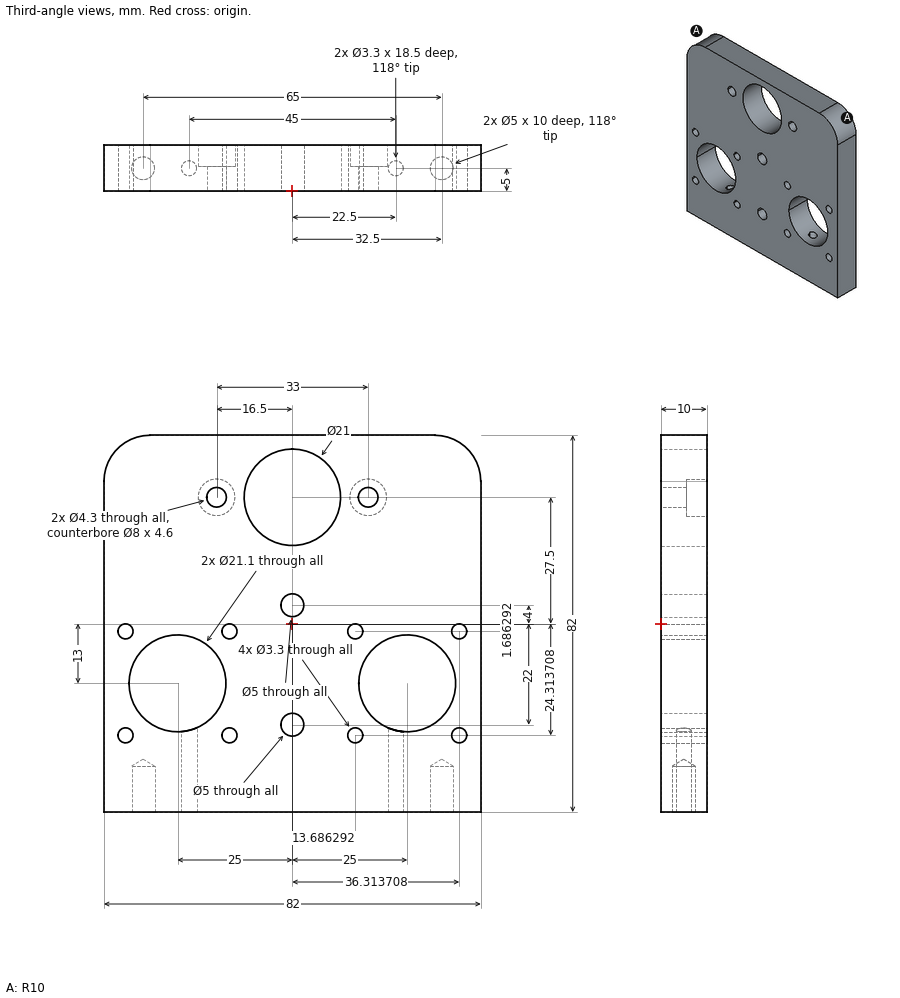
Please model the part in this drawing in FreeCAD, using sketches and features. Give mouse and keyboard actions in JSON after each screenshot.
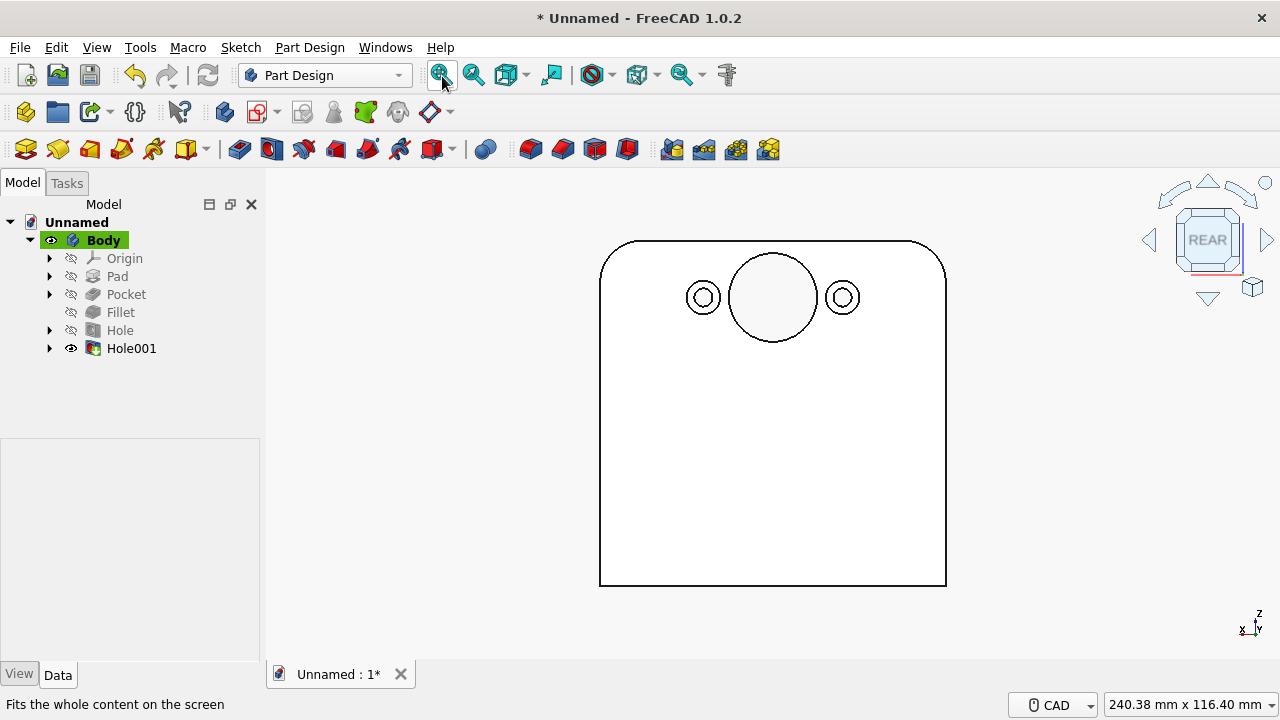
{"action": "left_click", "coordinate": [724, 462]}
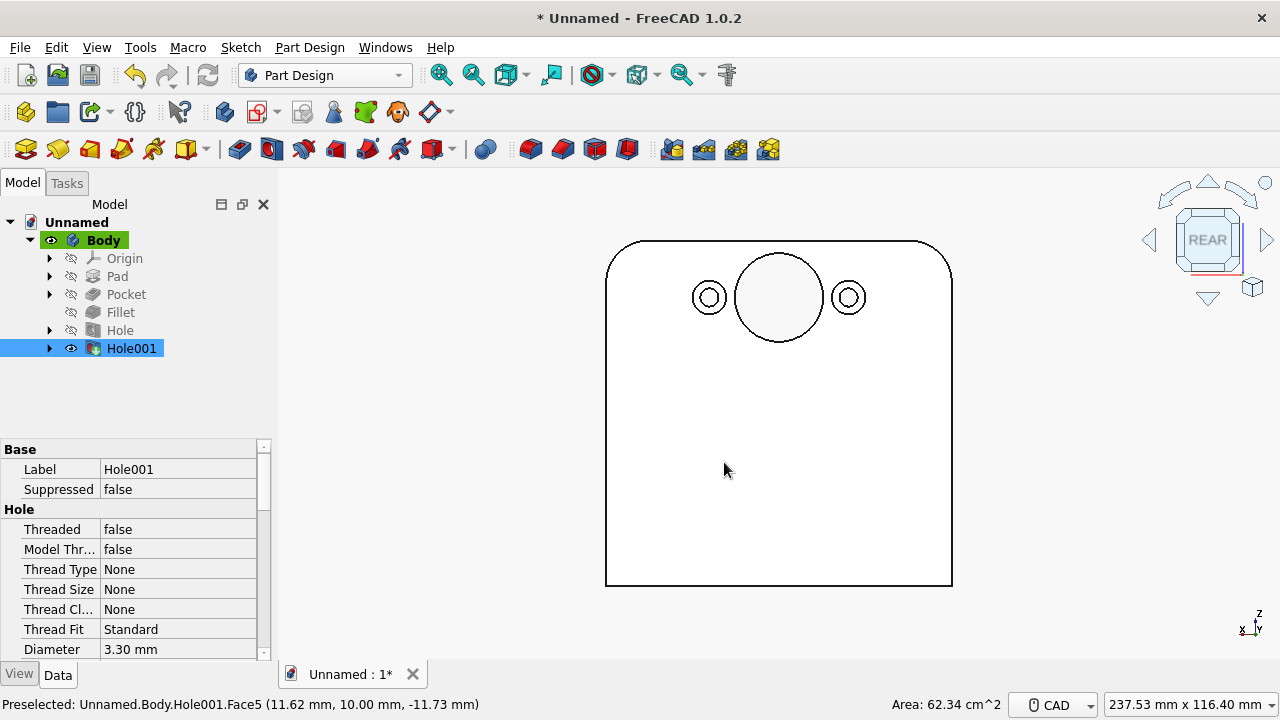
{"action": "left_click", "coordinate": [258, 112]}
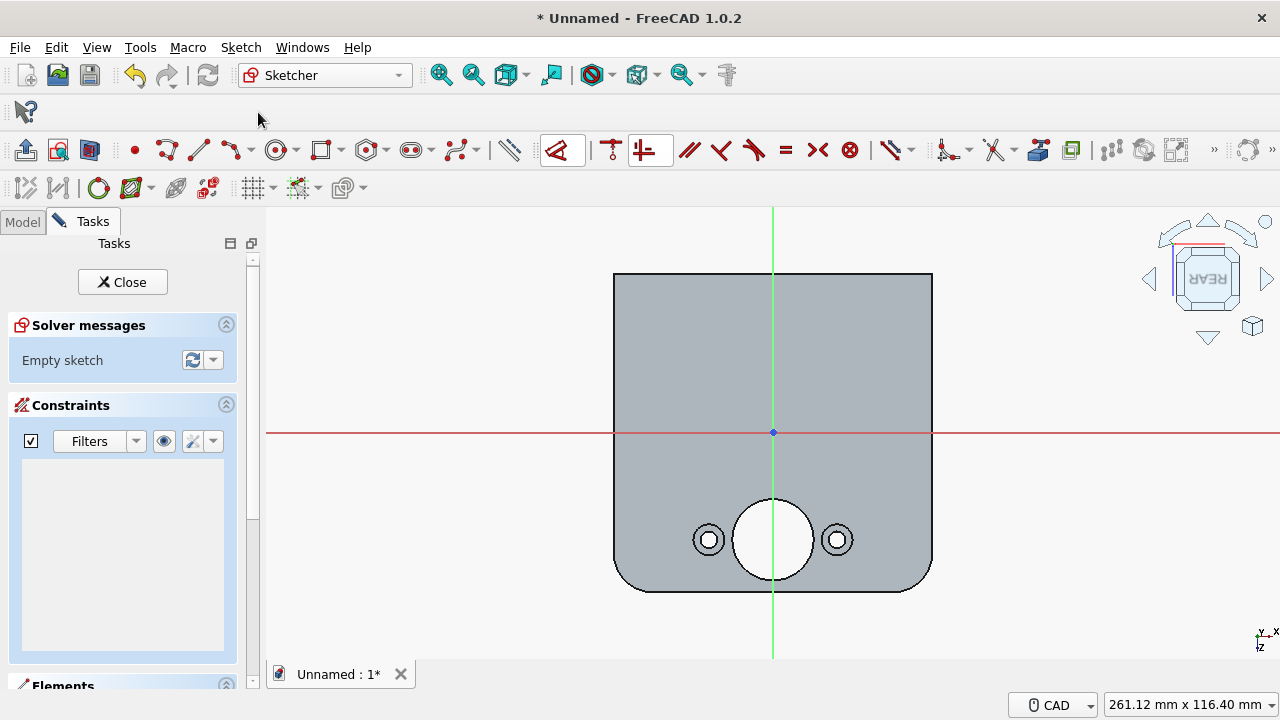
{"action": "scroll", "coordinate": [829, 350], "scroll_direction": "up", "scroll_amount": 4}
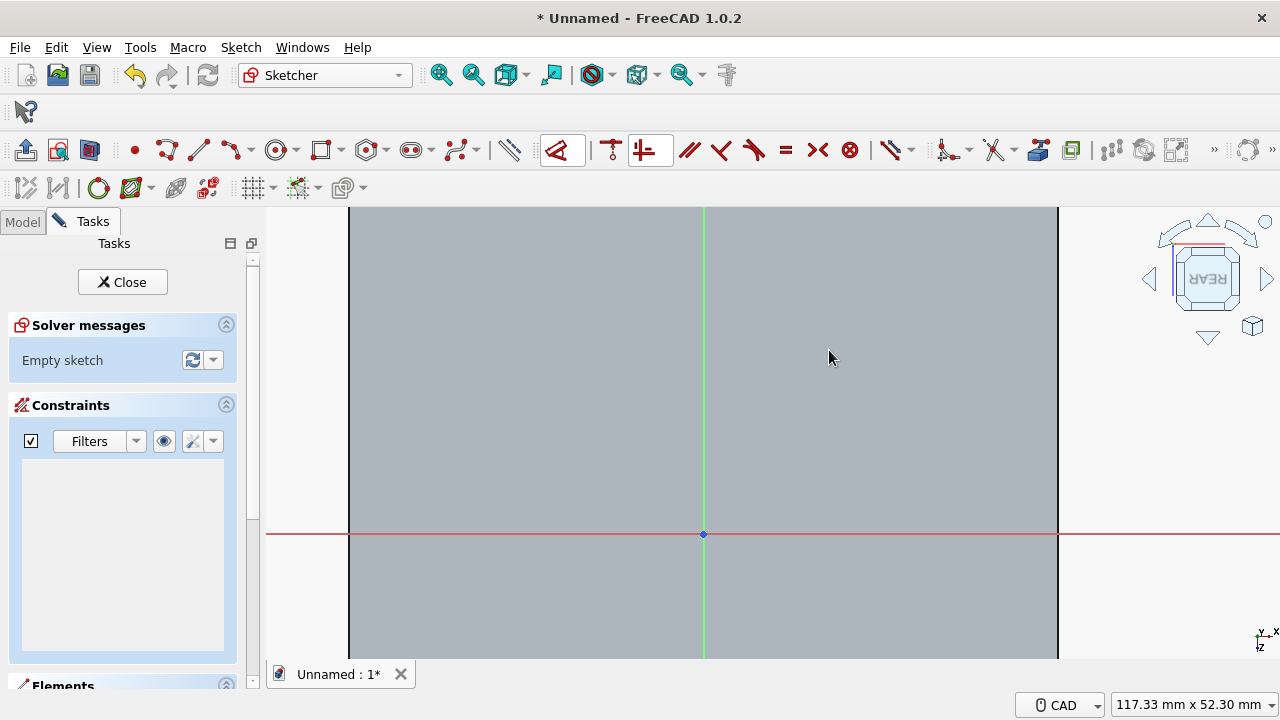
{"action": "left_click", "coordinate": [276, 150]}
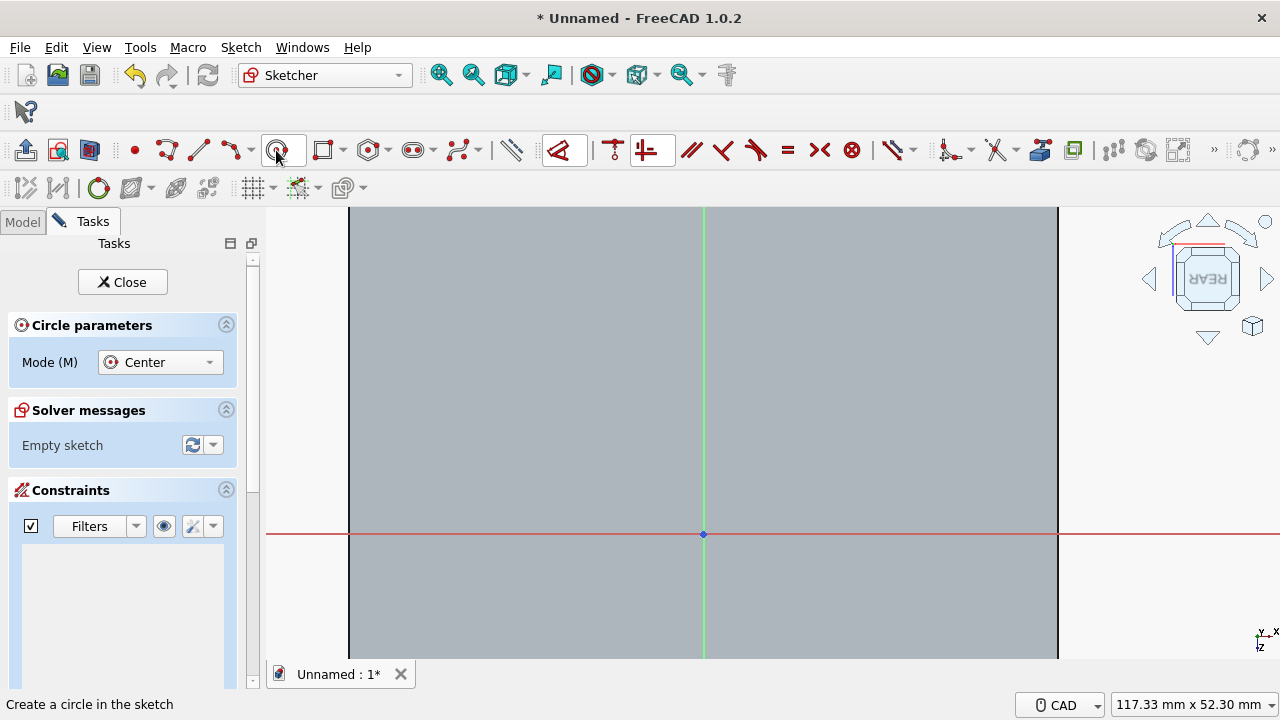
{"action": "left_click", "coordinate": [488, 422]}
{"action": "left_click", "coordinate": [552, 358]}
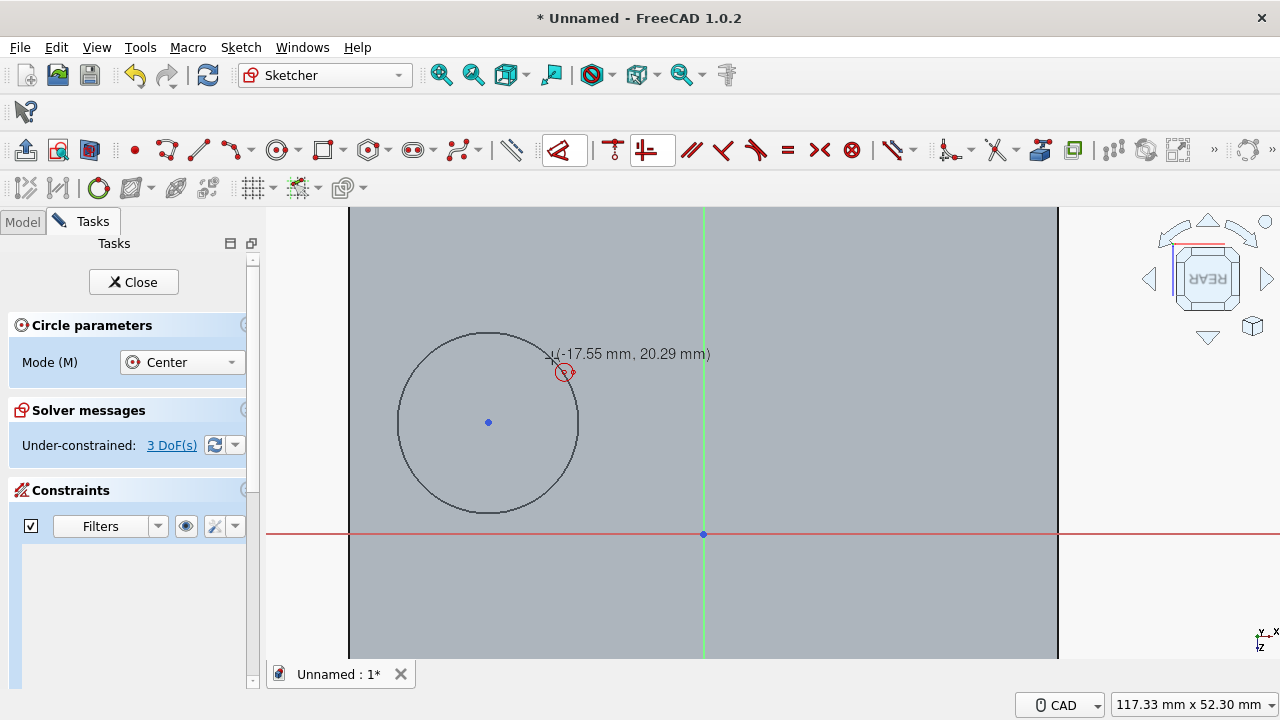
{"action": "left_click", "coordinate": [920, 422]}
{"action": "left_click", "coordinate": [984, 358]}
{"action": "key", "text": "Escape"}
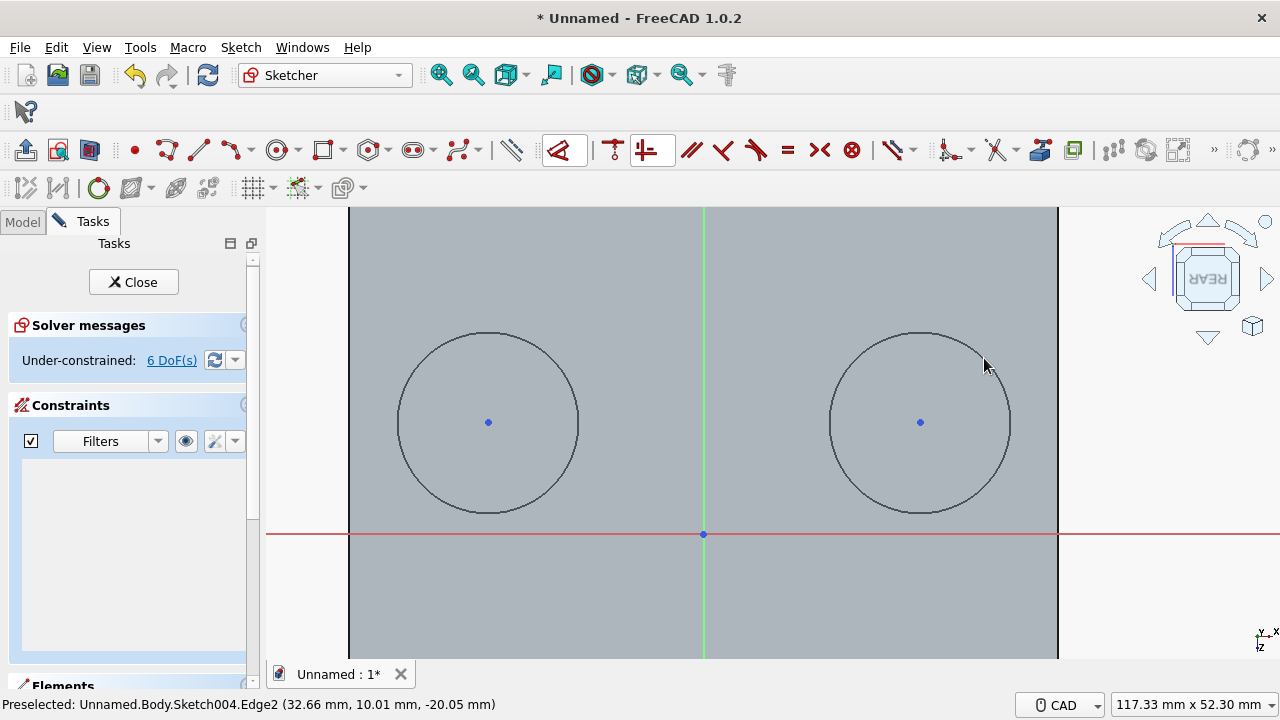
{"action": "left_click", "coordinate": [552, 359]}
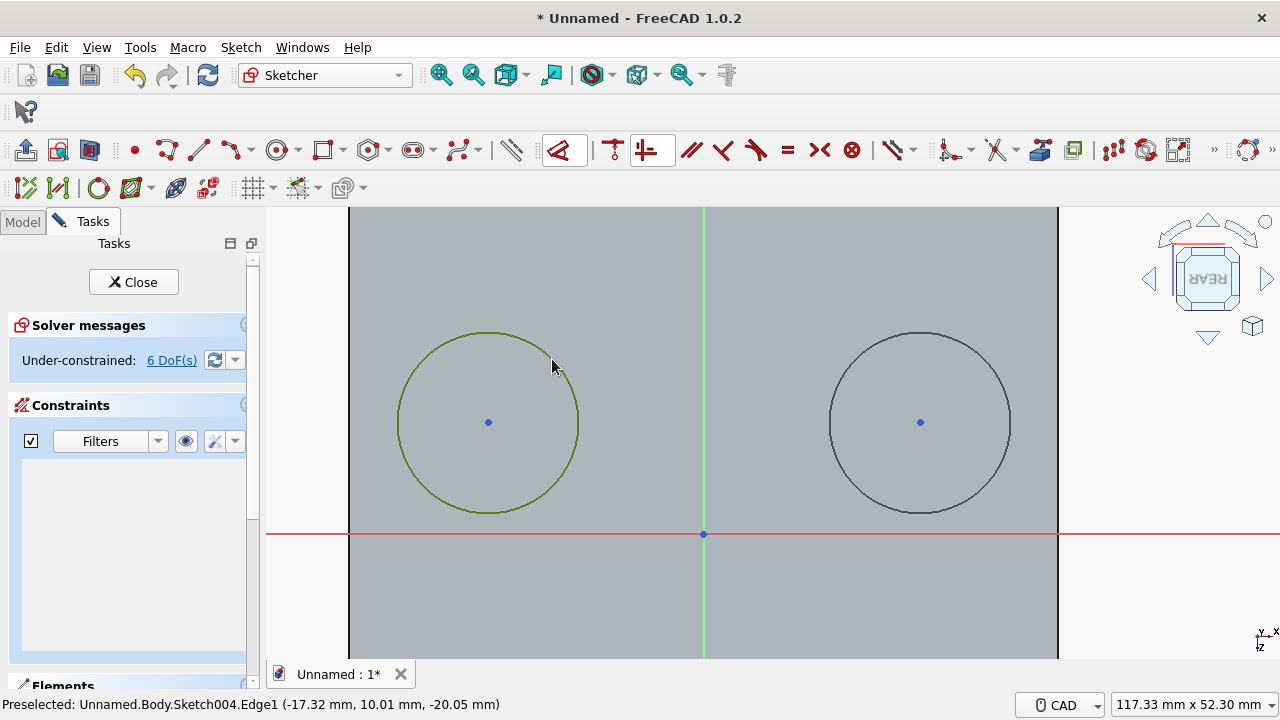
{"action": "left_click", "coordinate": [984, 359]}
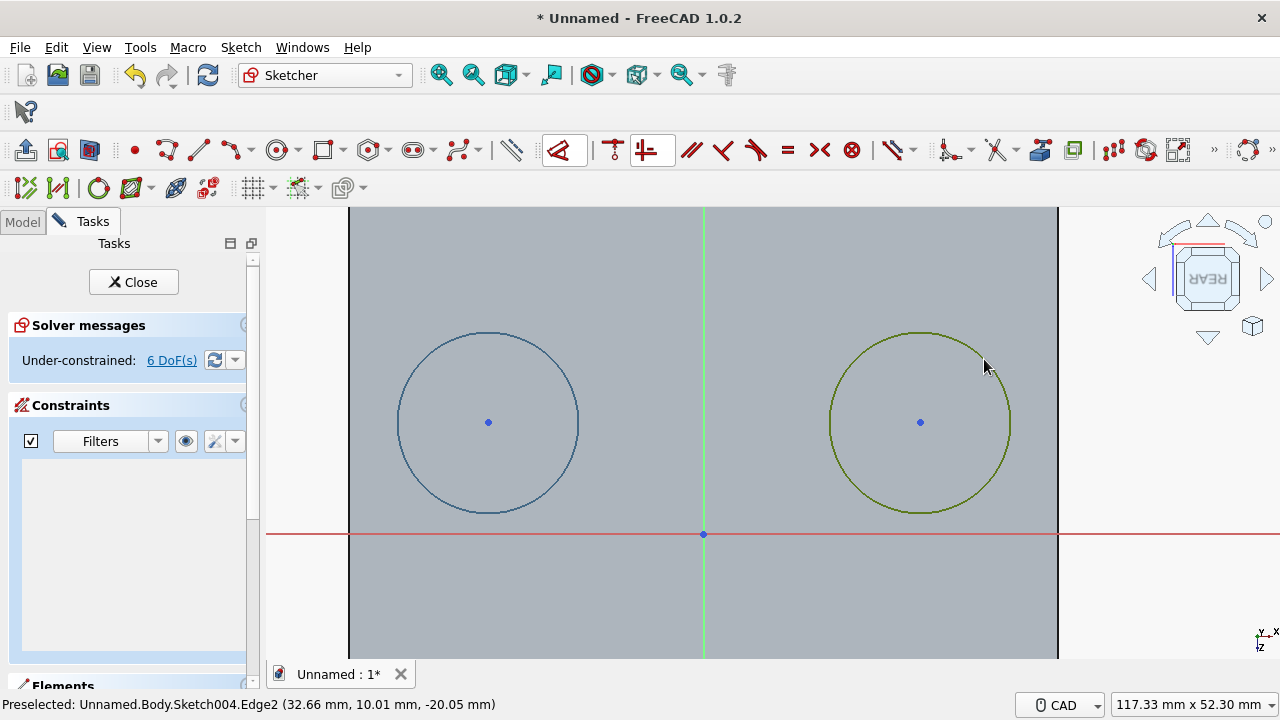
{"action": "left_click", "coordinate": [788, 150]}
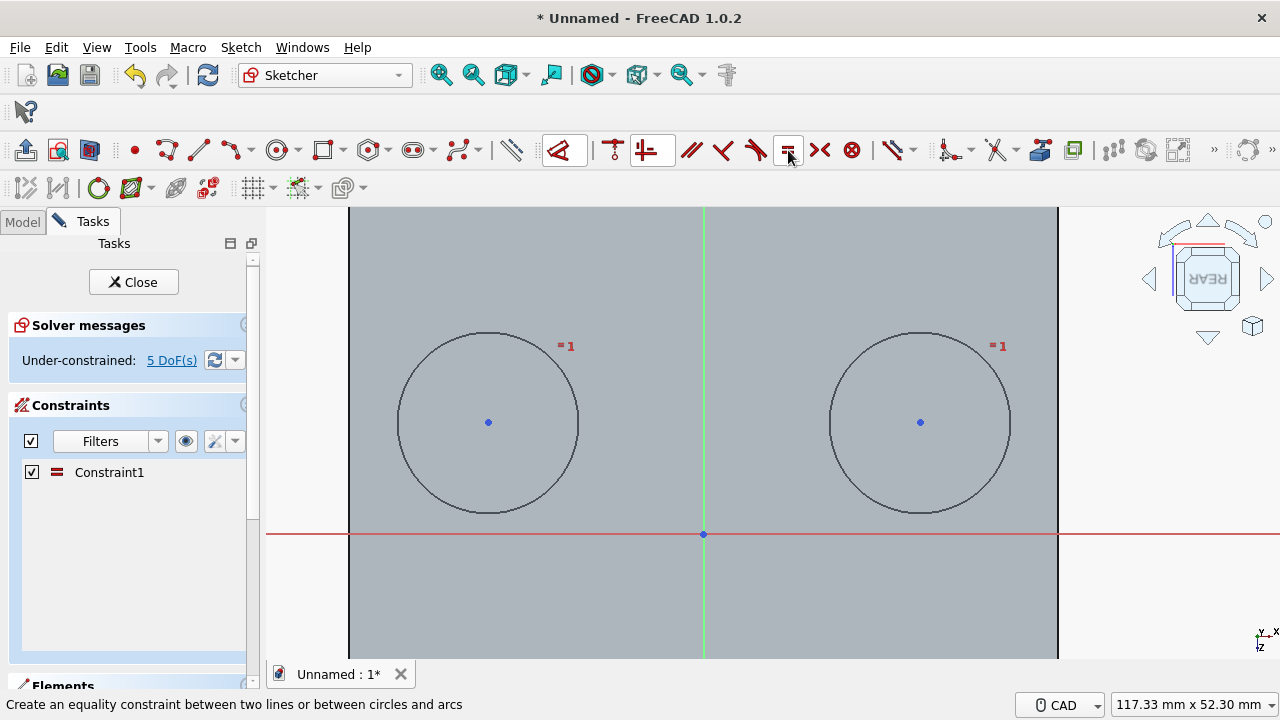
{"action": "left_click", "coordinate": [552, 359]}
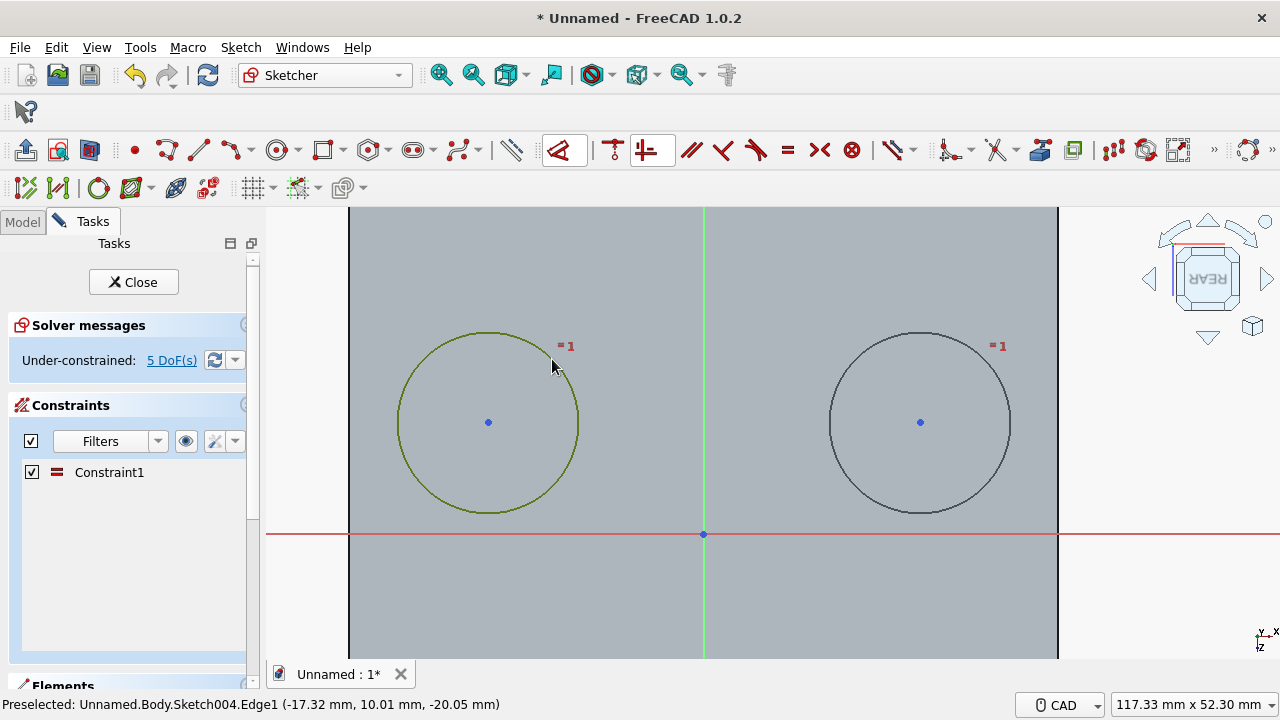
{"action": "key", "text": "k o"}